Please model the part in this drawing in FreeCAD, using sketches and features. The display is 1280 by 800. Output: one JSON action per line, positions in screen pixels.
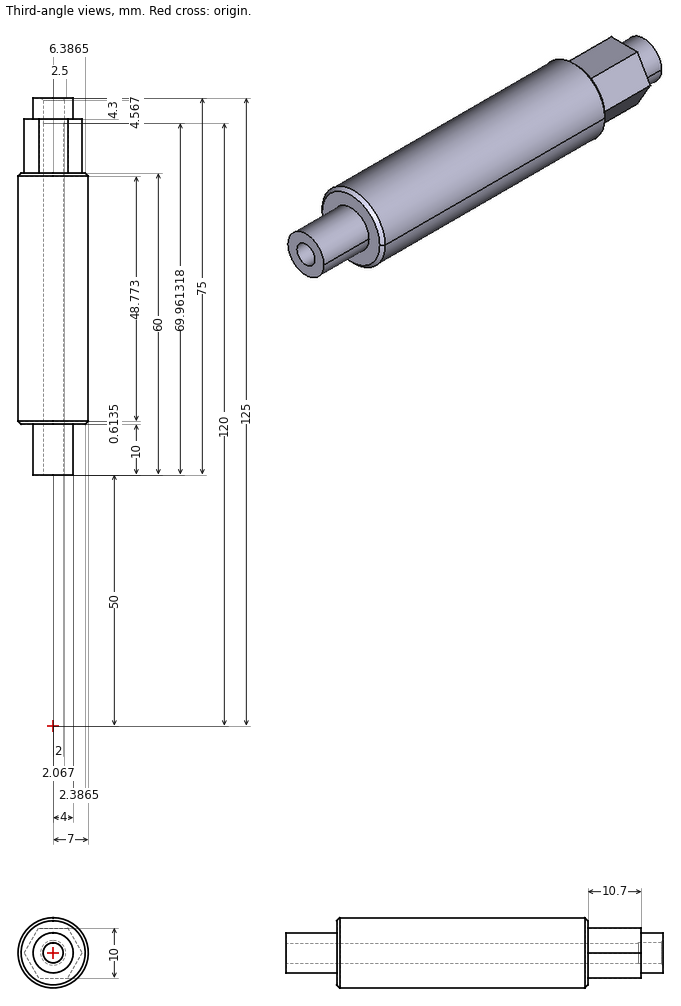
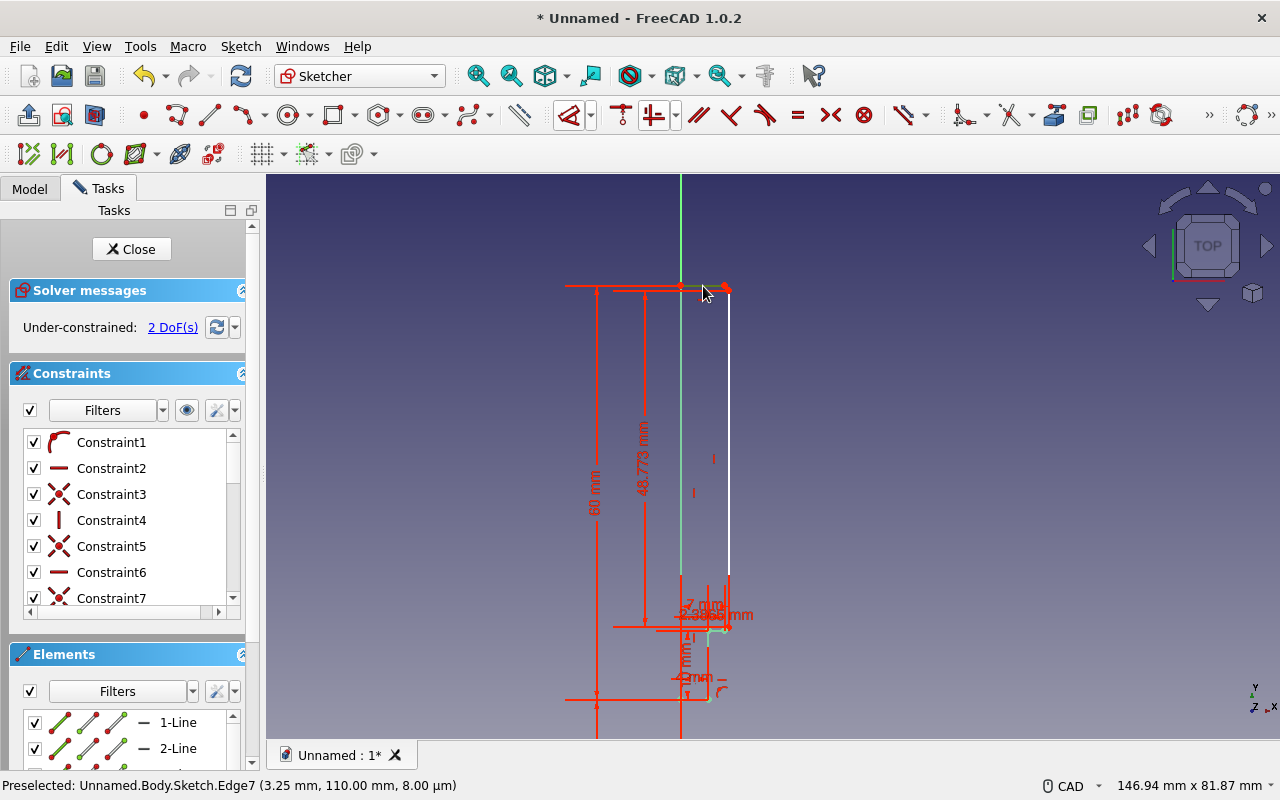
{"action": "key", "text": "l"}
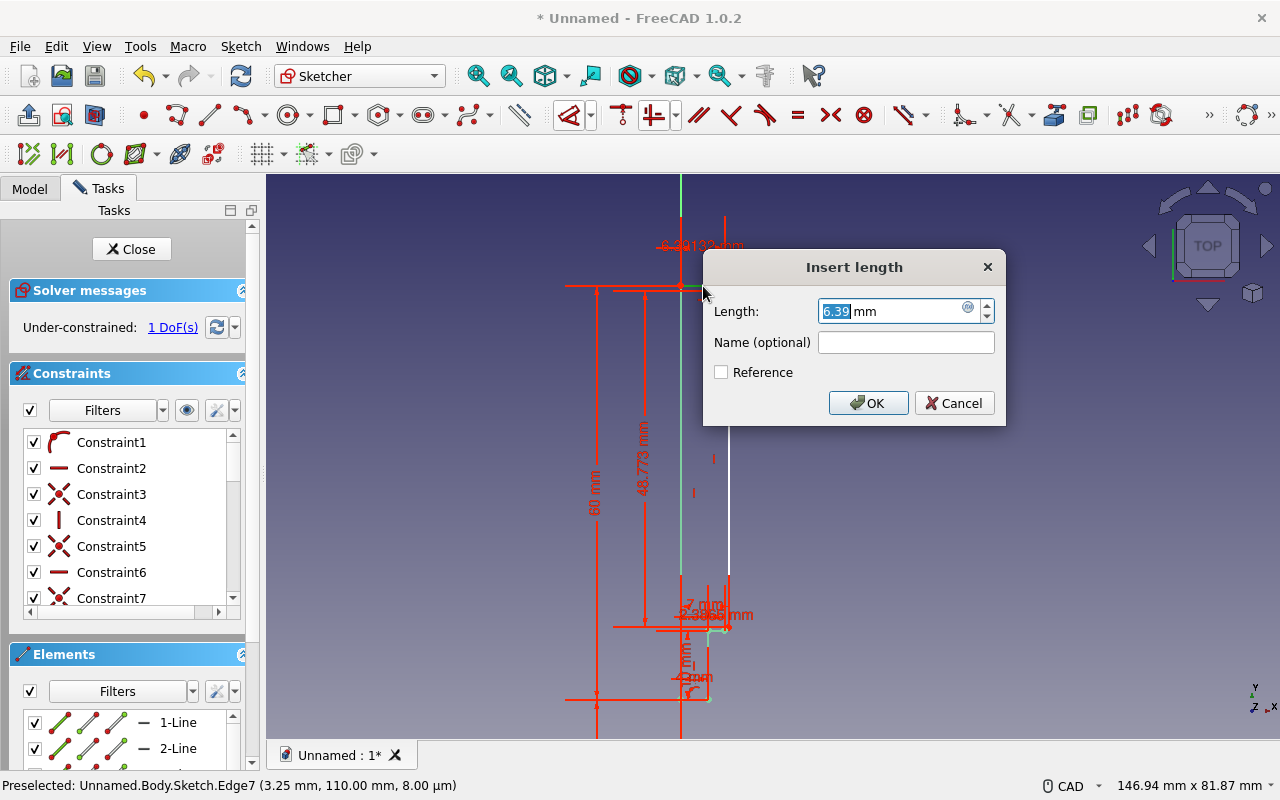
{"action": "type", "text": "6.3865"}
{"action": "key", "text": "Return"}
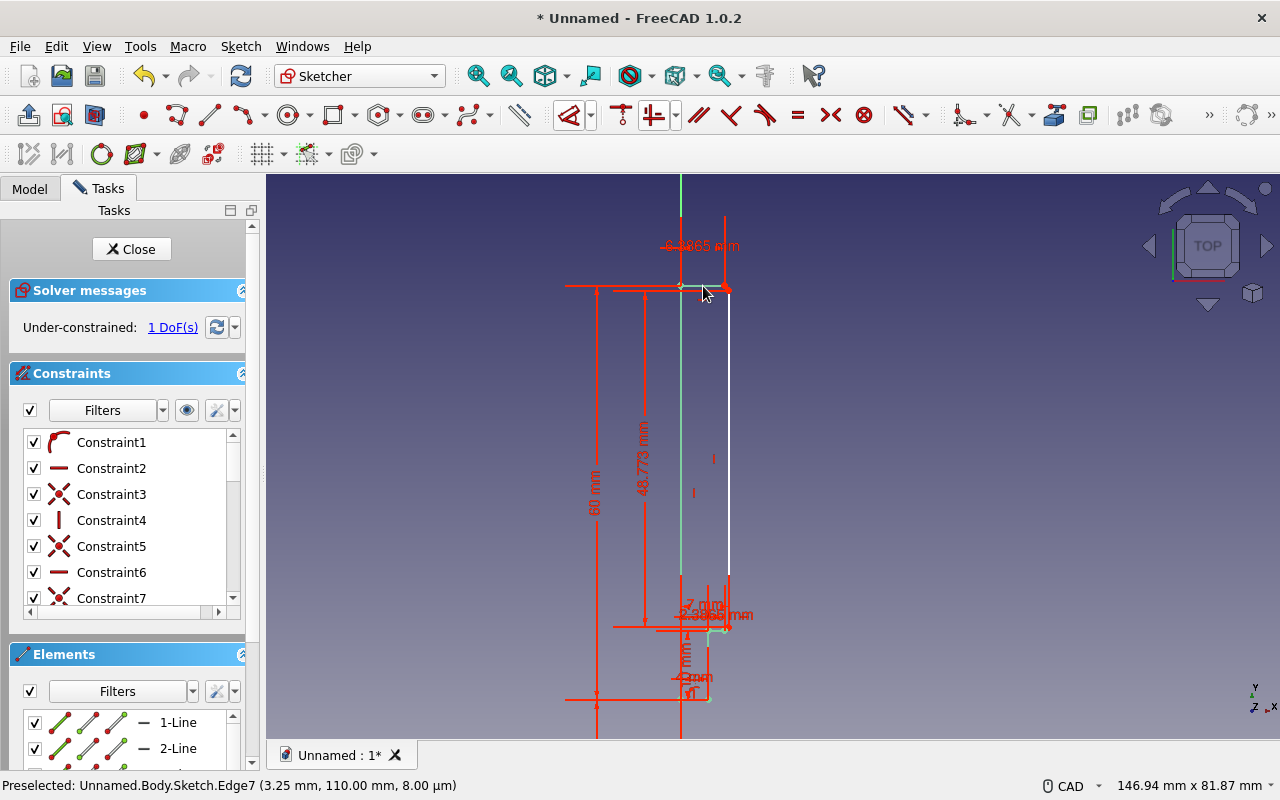
{"action": "scroll", "coordinate": [727, 629], "scroll_direction": "up", "scroll_amount": 12}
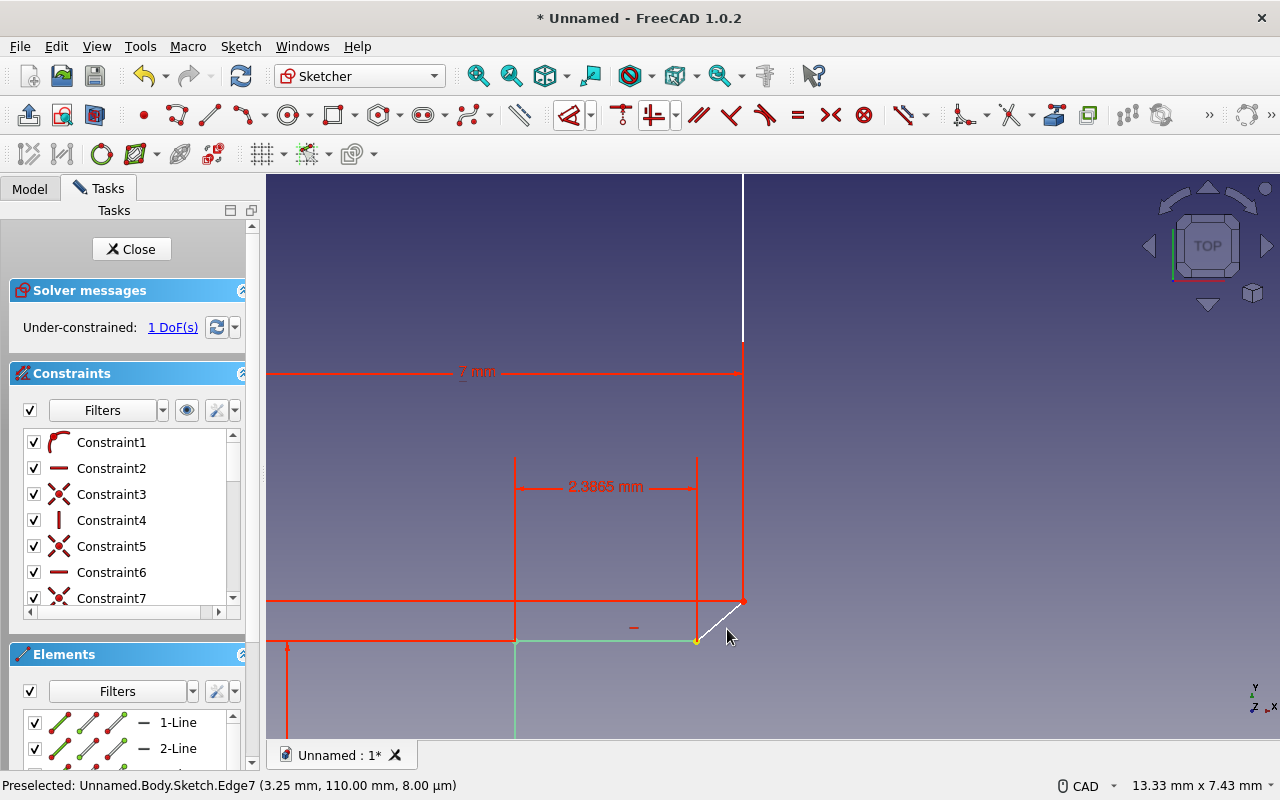
{"action": "left_click", "coordinate": [720, 621]}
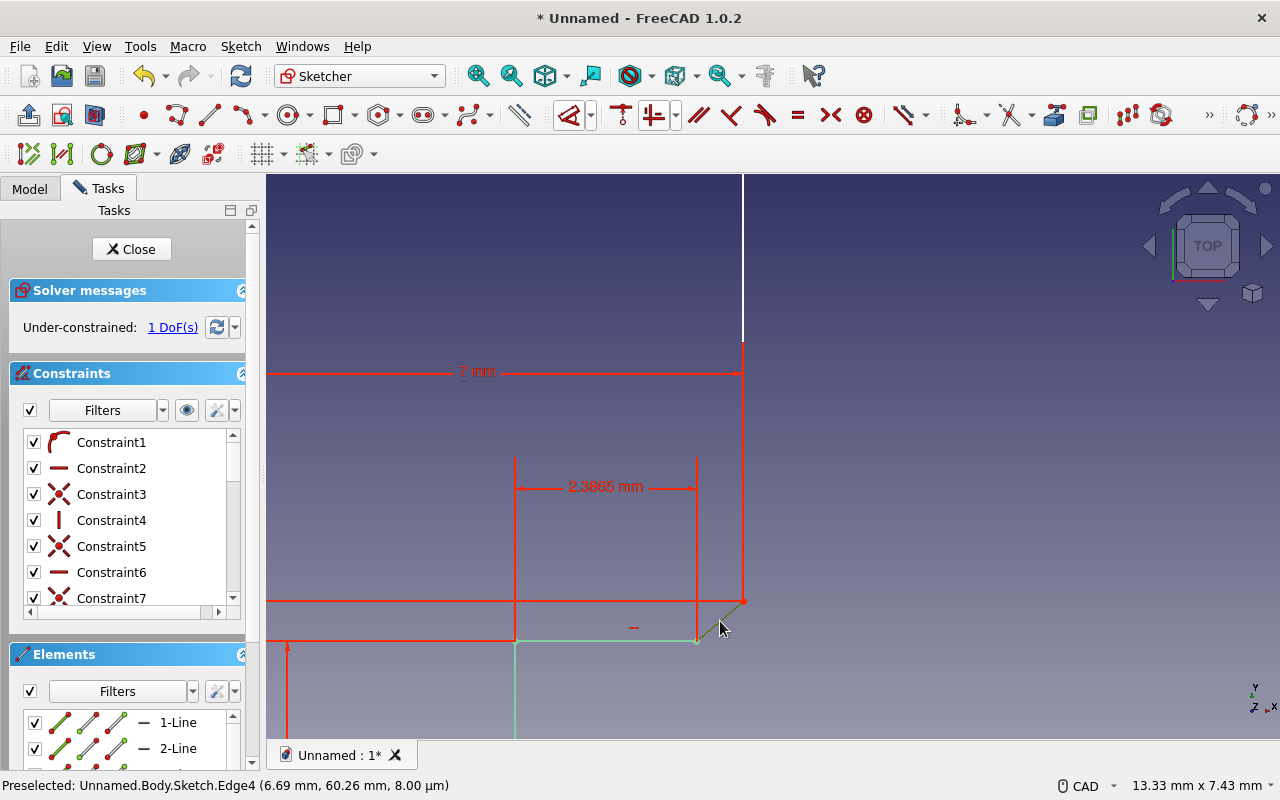
{"action": "key", "text": "i"}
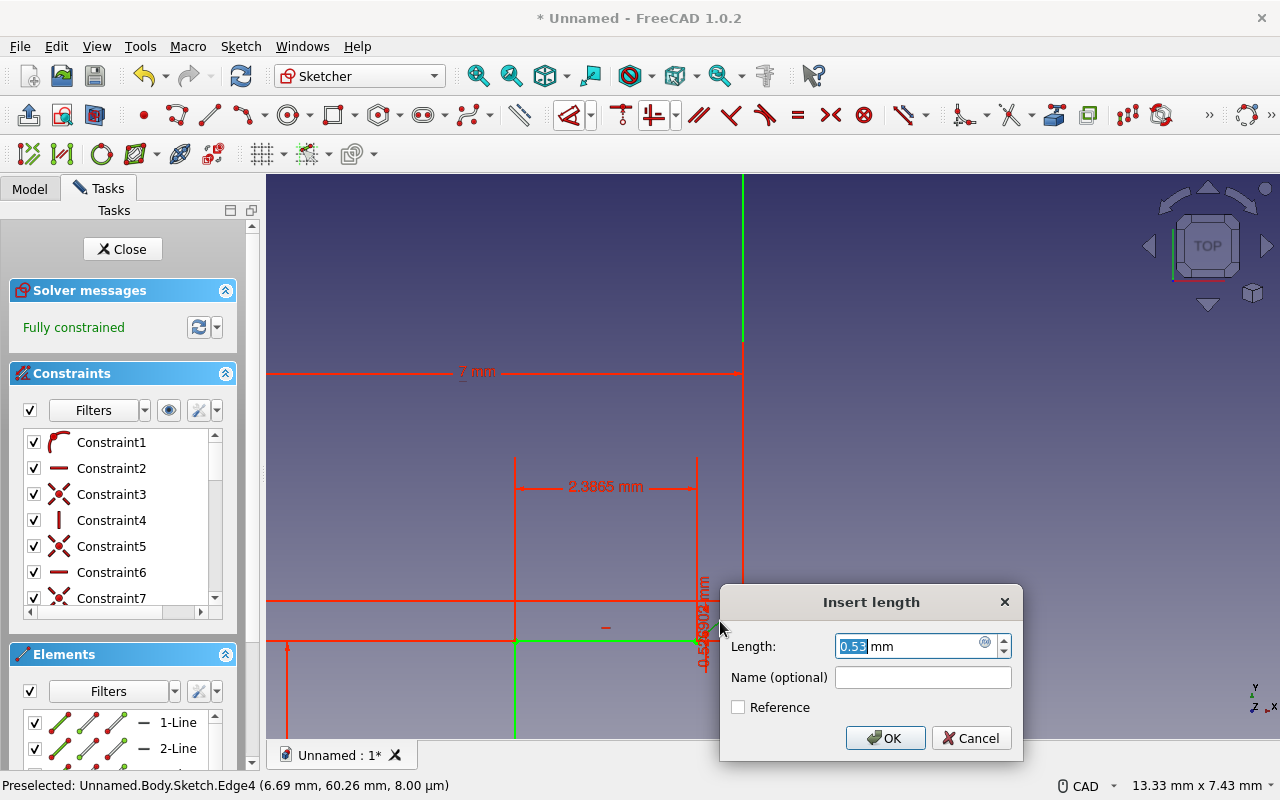
{"action": "type", "text": "0.6135"}
{"action": "key", "text": "Return"}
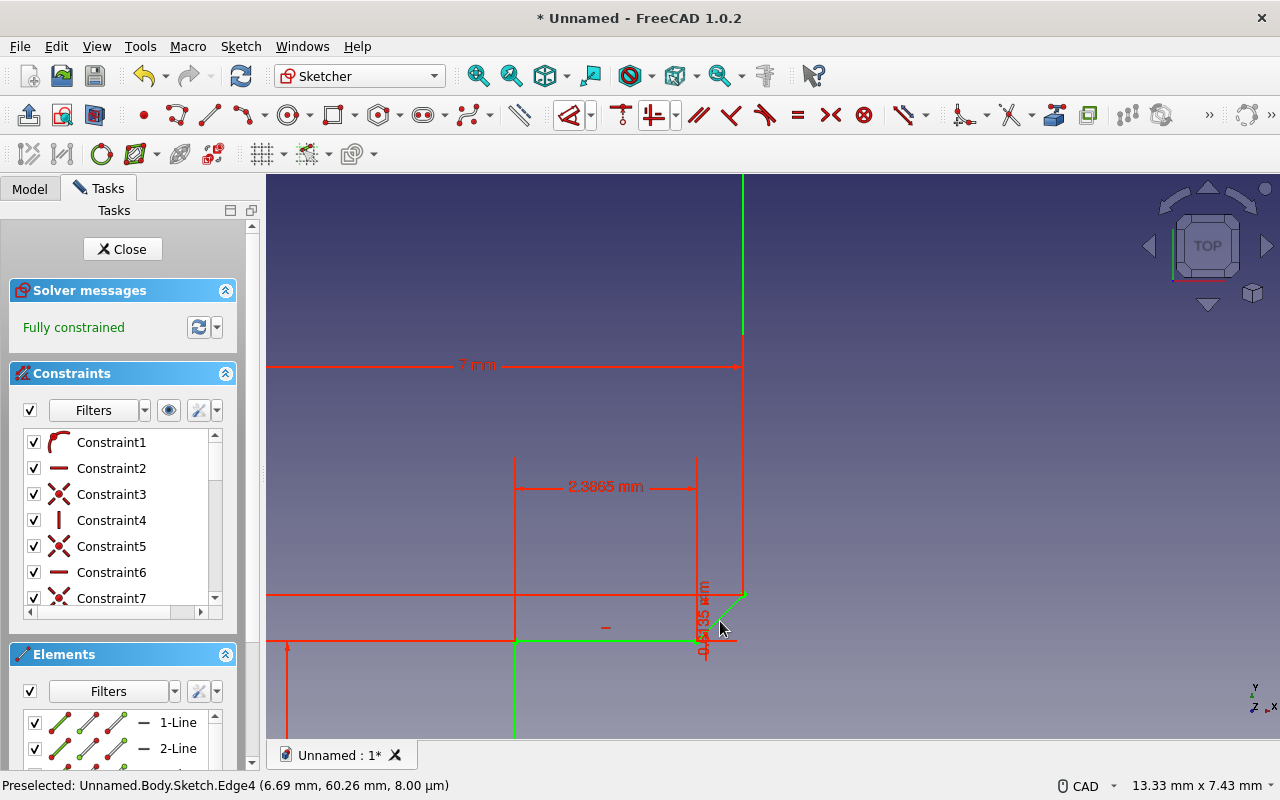
{"action": "left_click", "coordinate": [123, 249]}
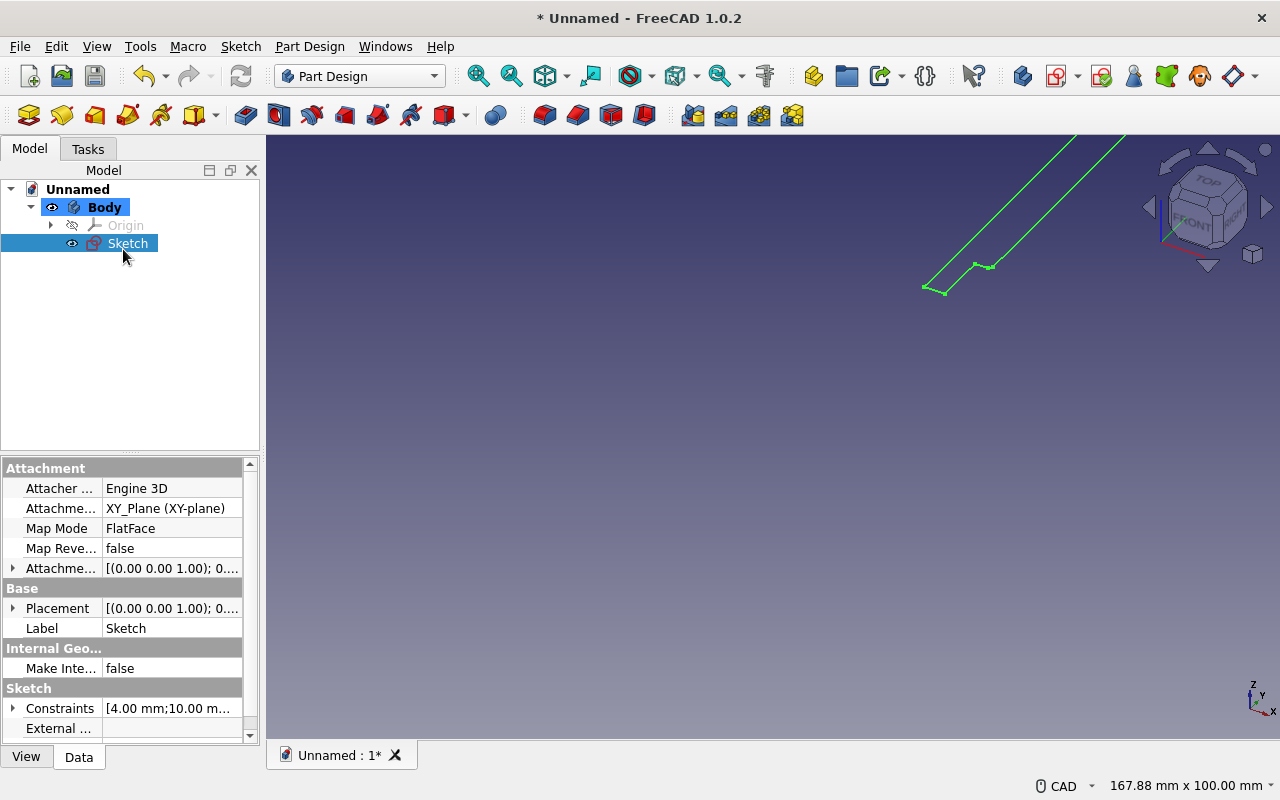
{"action": "left_click", "coordinate": [62, 116]}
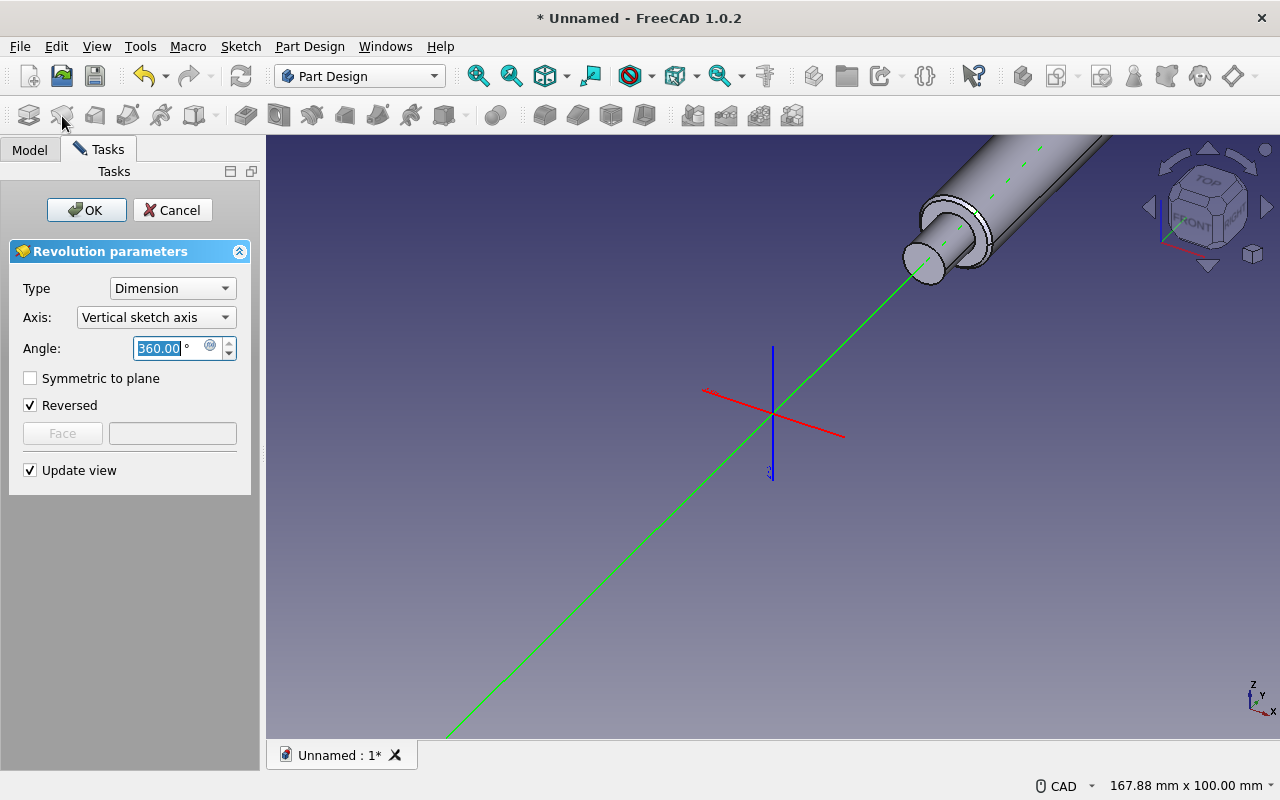
{"action": "left_click", "coordinate": [87, 210]}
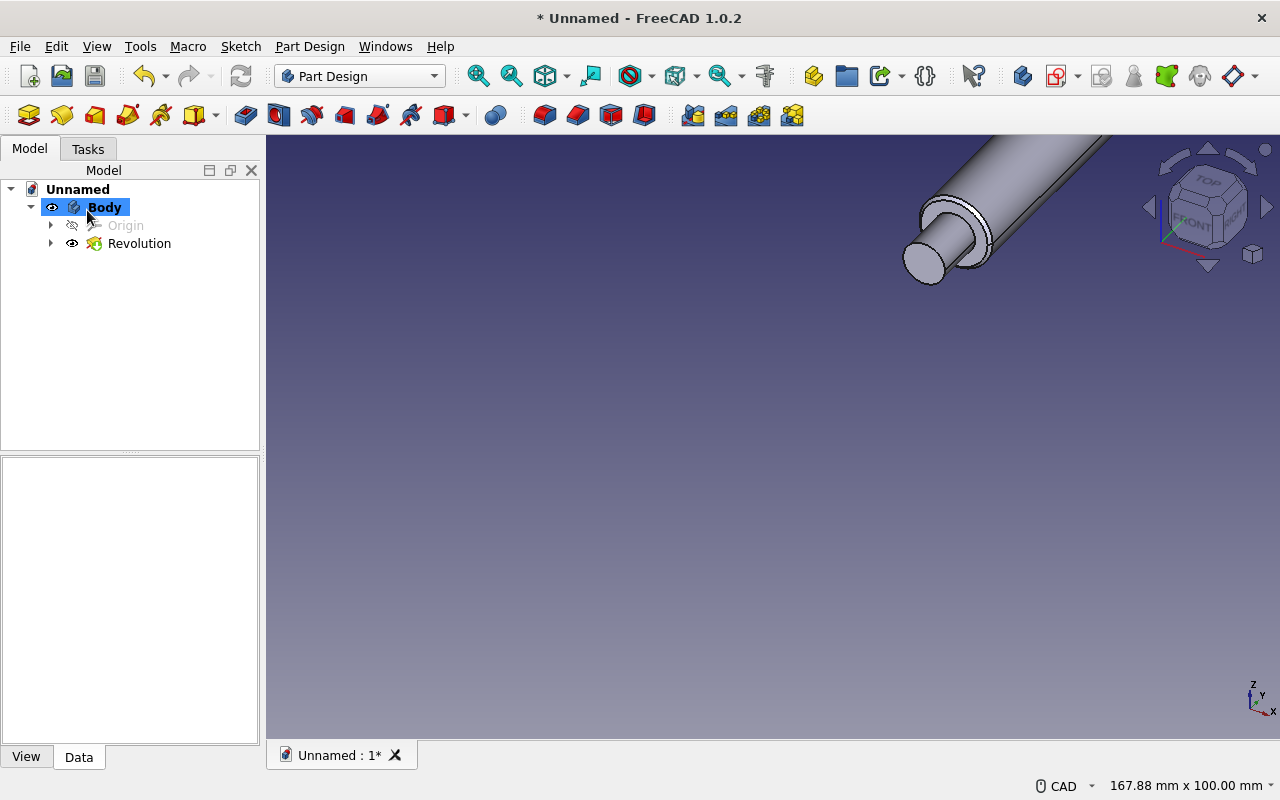
{"action": "left_click", "coordinate": [479, 76]}